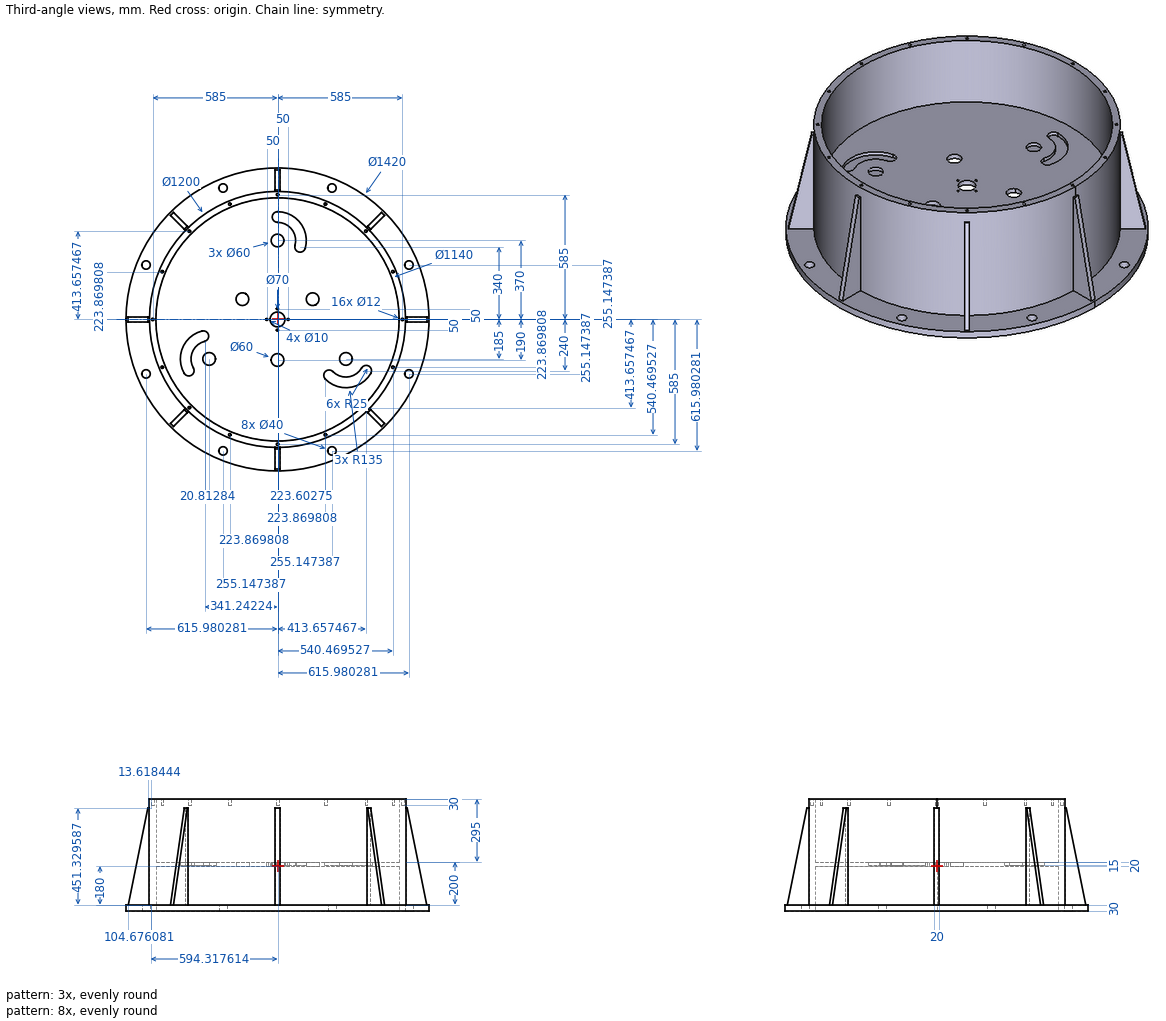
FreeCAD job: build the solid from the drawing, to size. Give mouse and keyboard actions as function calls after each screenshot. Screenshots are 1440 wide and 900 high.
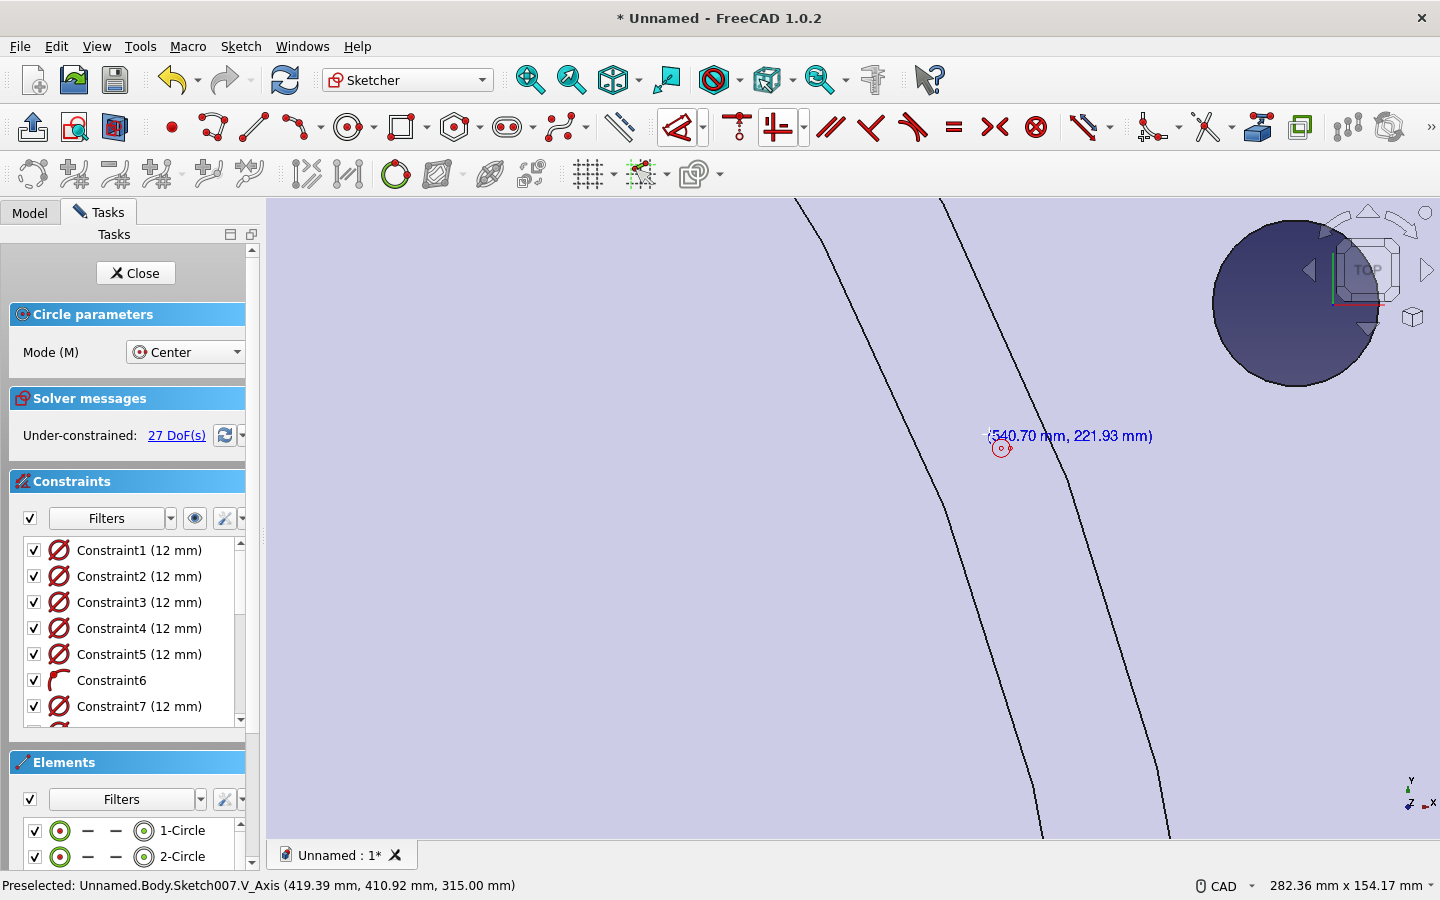
scroll(989, 434, down, 12)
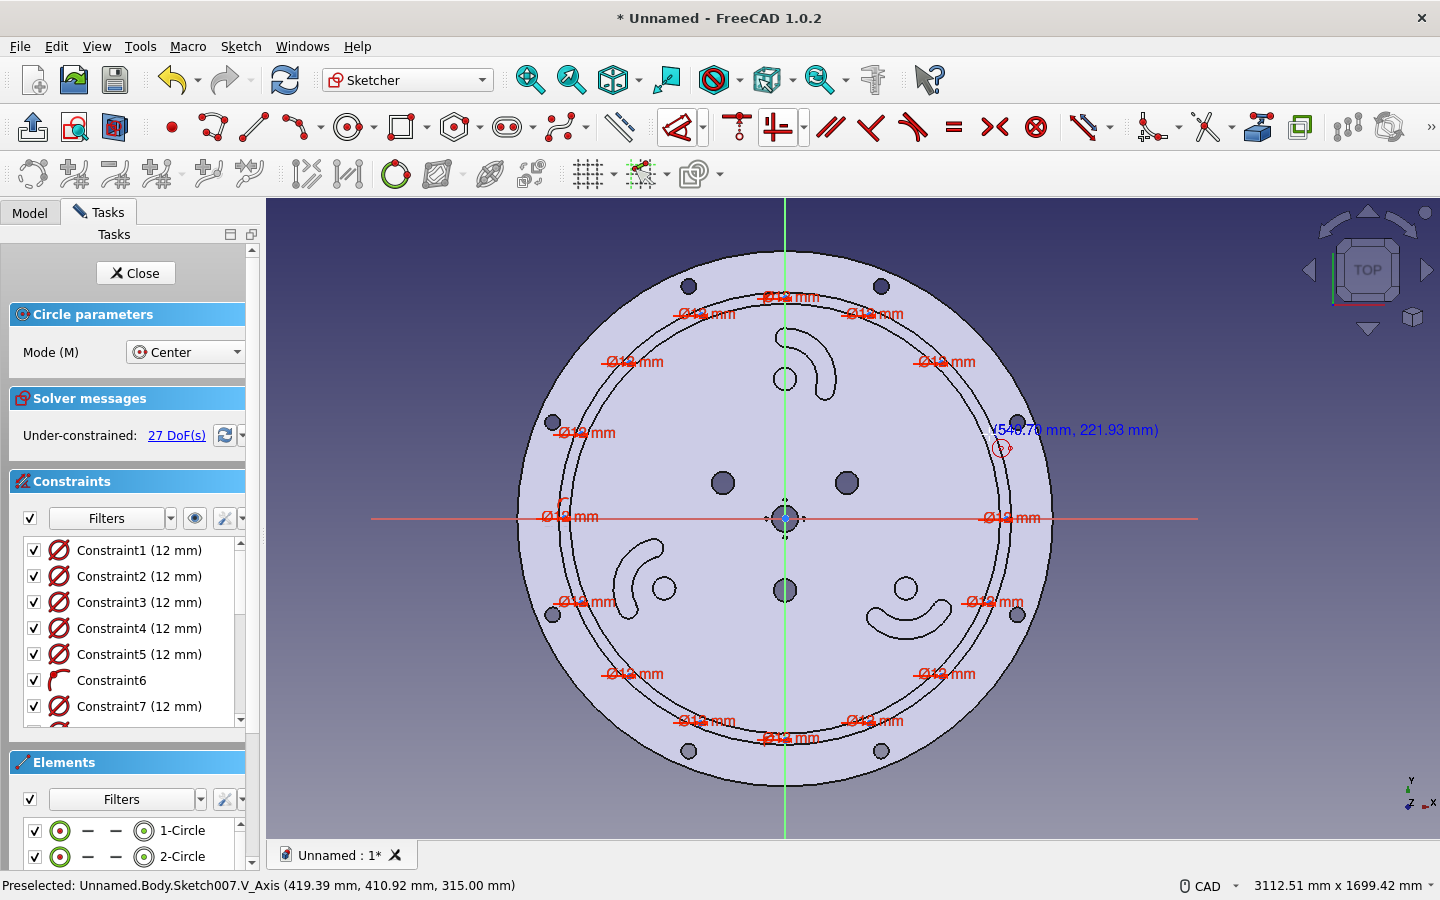
click(989, 434)
move(991, 433)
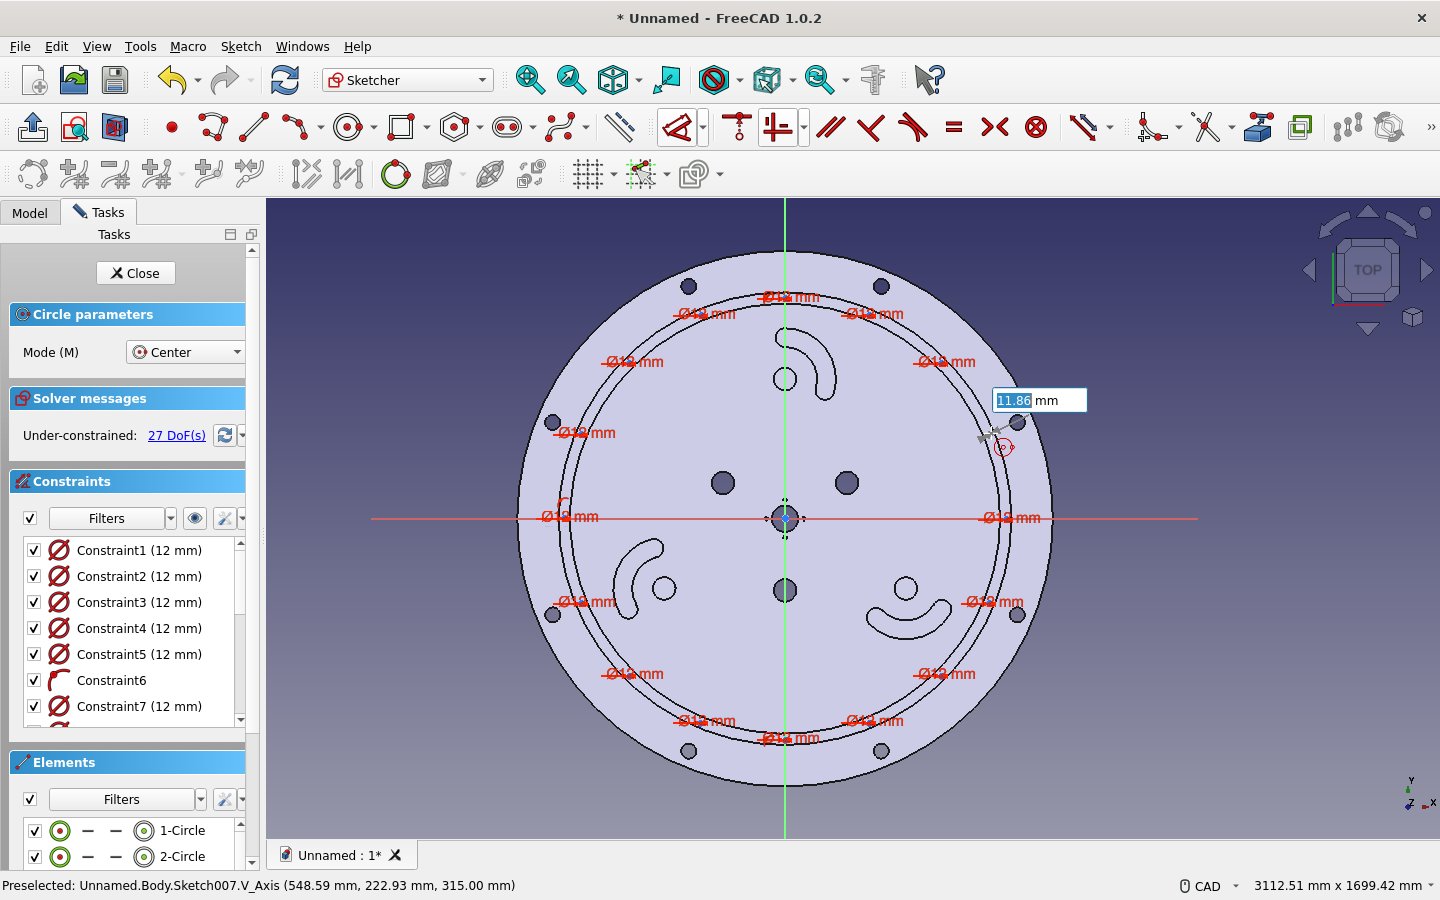
text(12)
key(Return)
key(Escape)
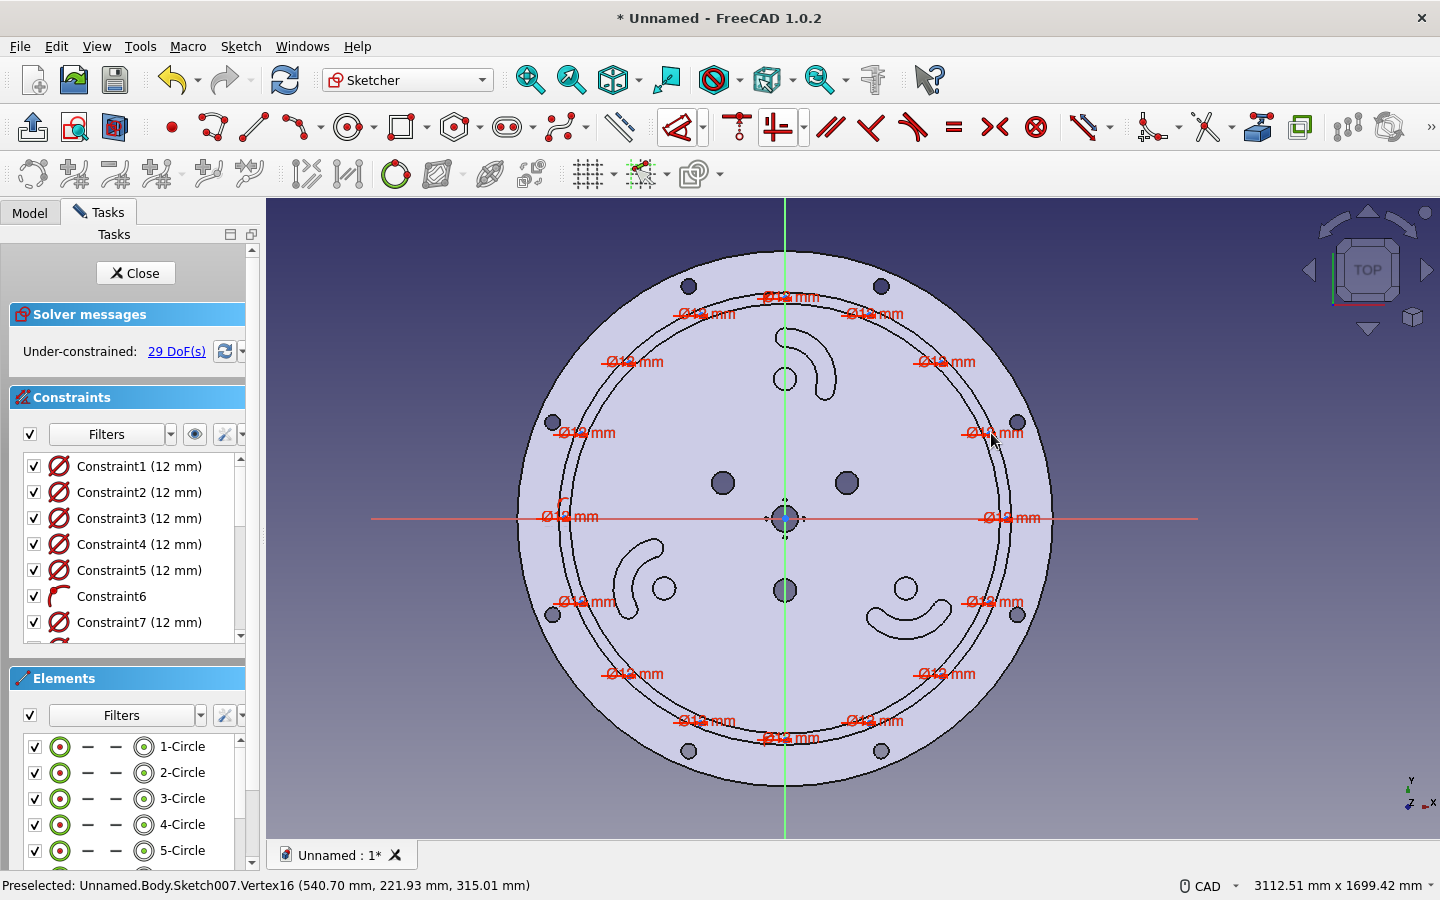
click(1006, 520)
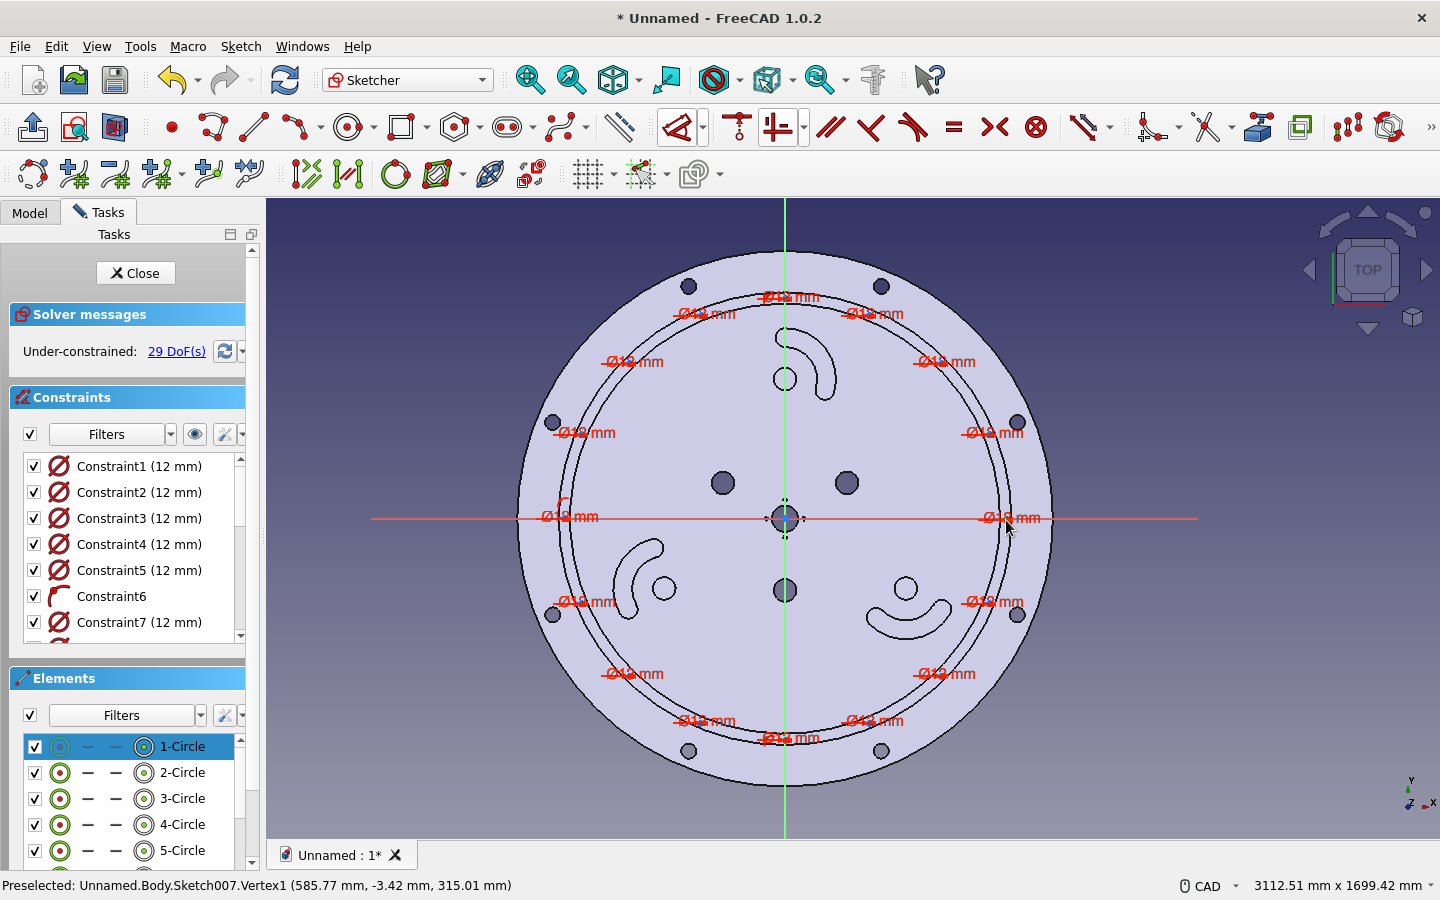
click(434, 519)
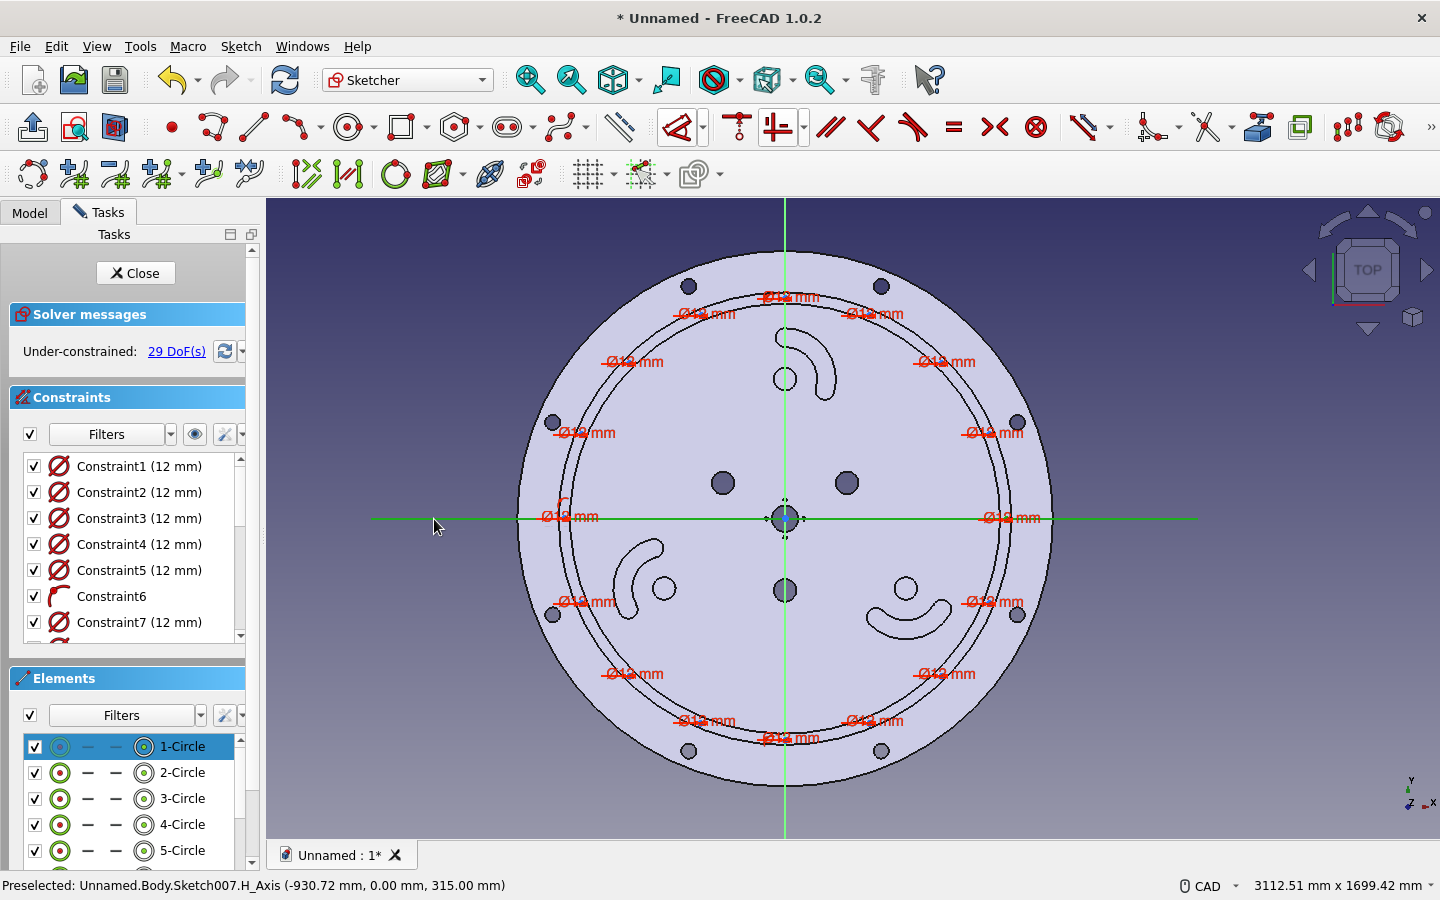
click(737, 128)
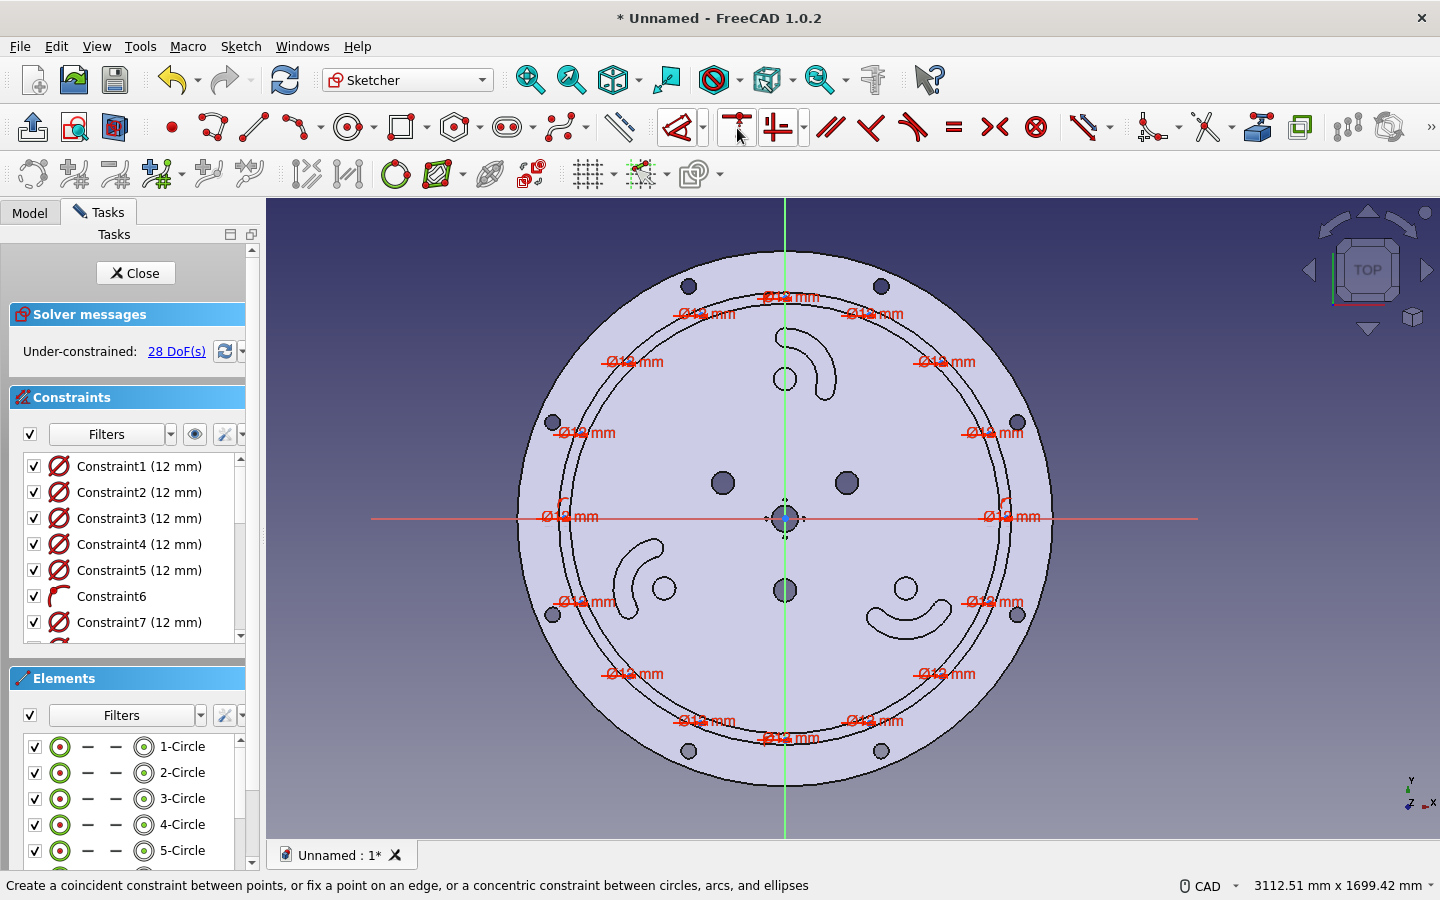
click(869, 723)